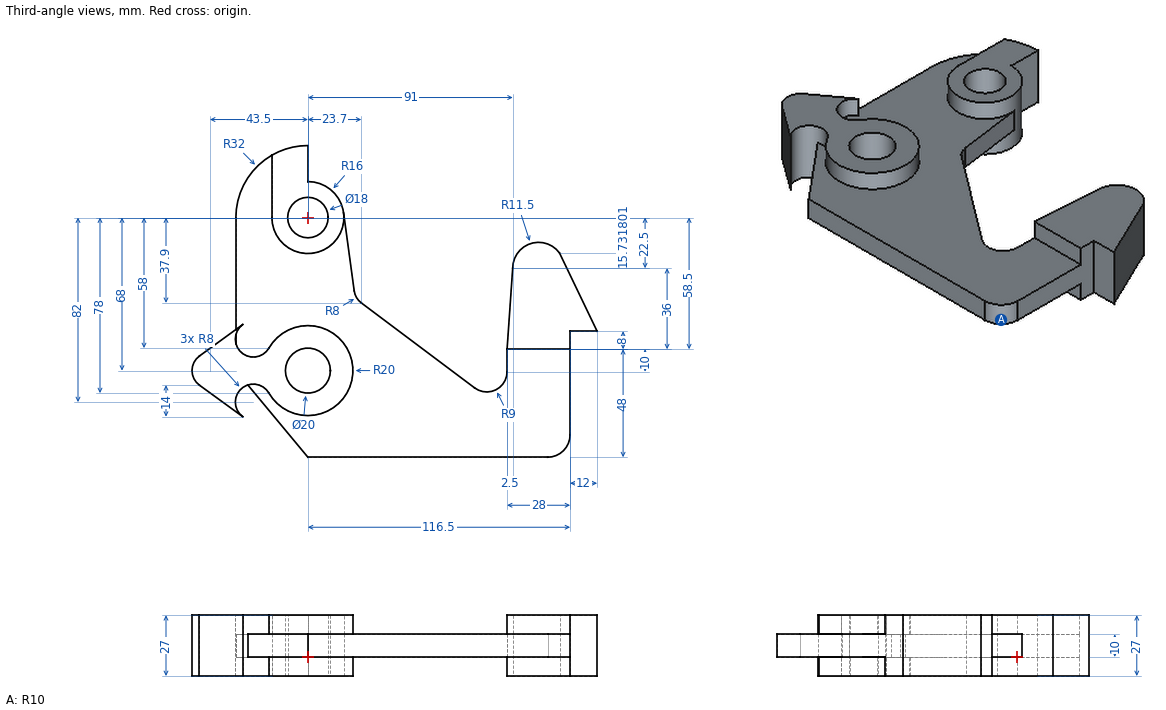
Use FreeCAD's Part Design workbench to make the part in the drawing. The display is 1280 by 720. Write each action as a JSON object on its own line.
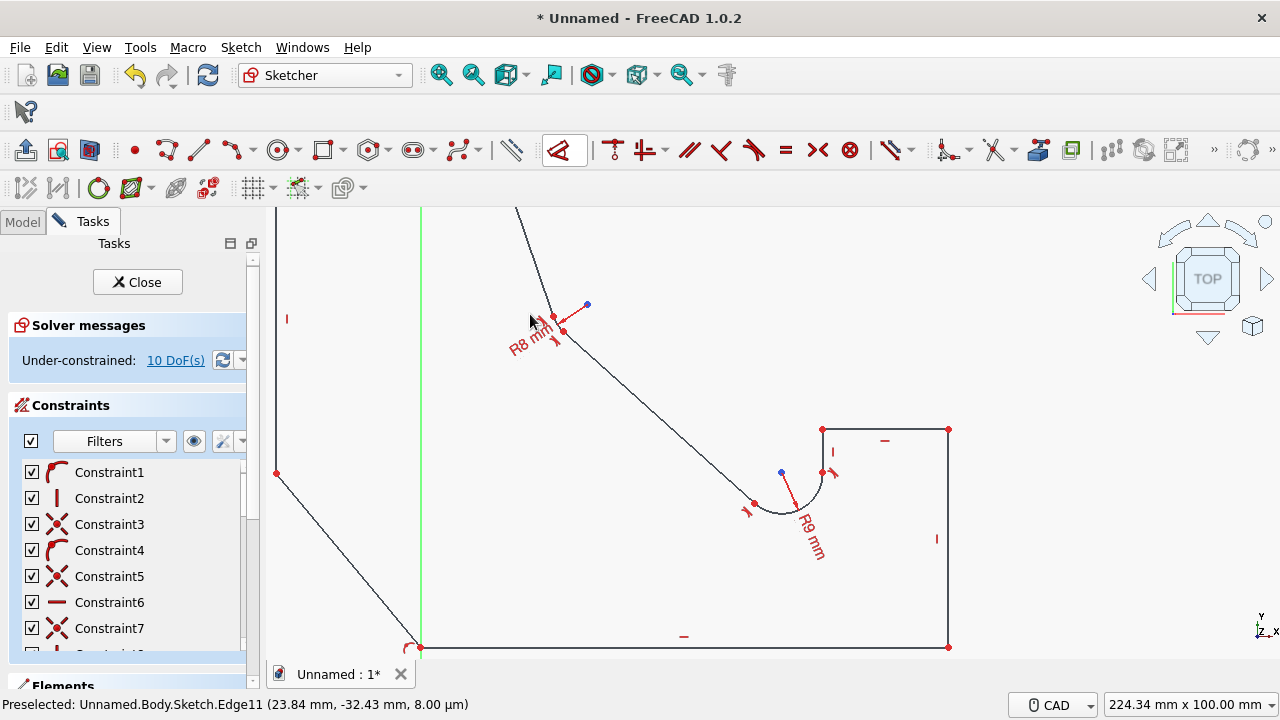
{"action": "scroll", "coordinate": [780, 515], "scroll_direction": "down", "scroll_amount": 4}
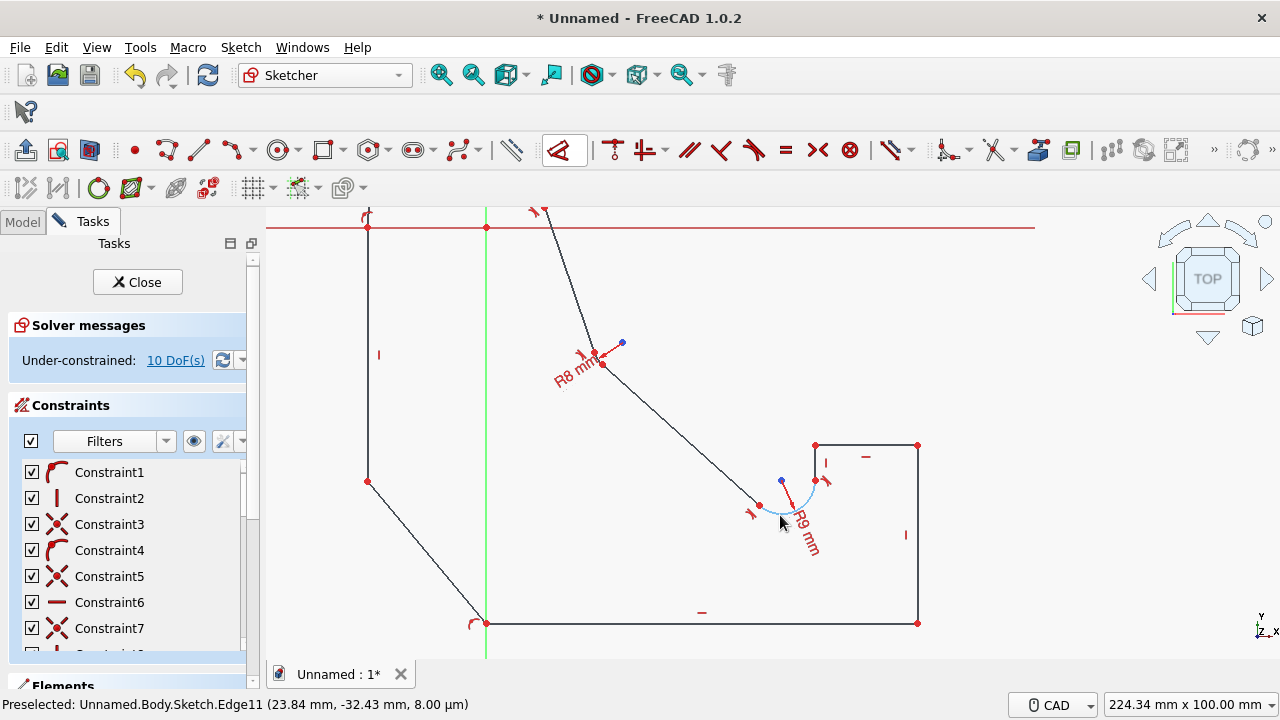
{"action": "scroll", "coordinate": [645, 336], "scroll_direction": "up", "scroll_amount": 2}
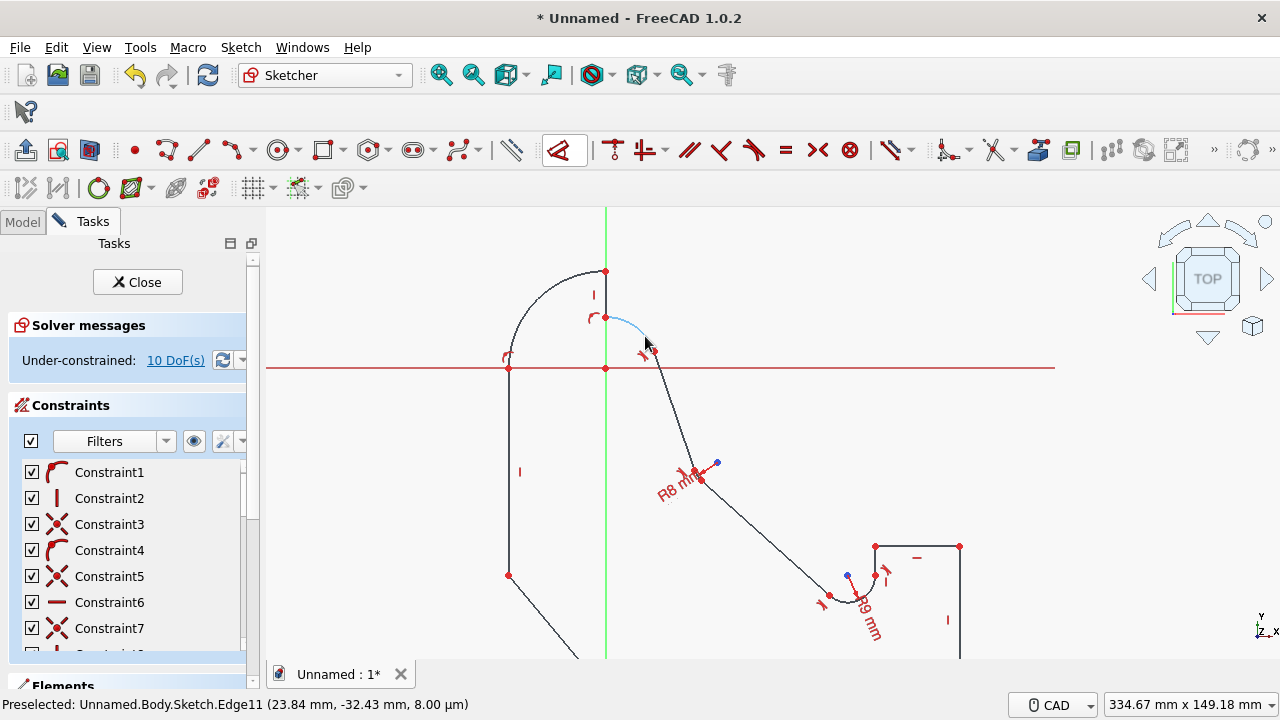
{"action": "left_click", "coordinate": [645, 335]}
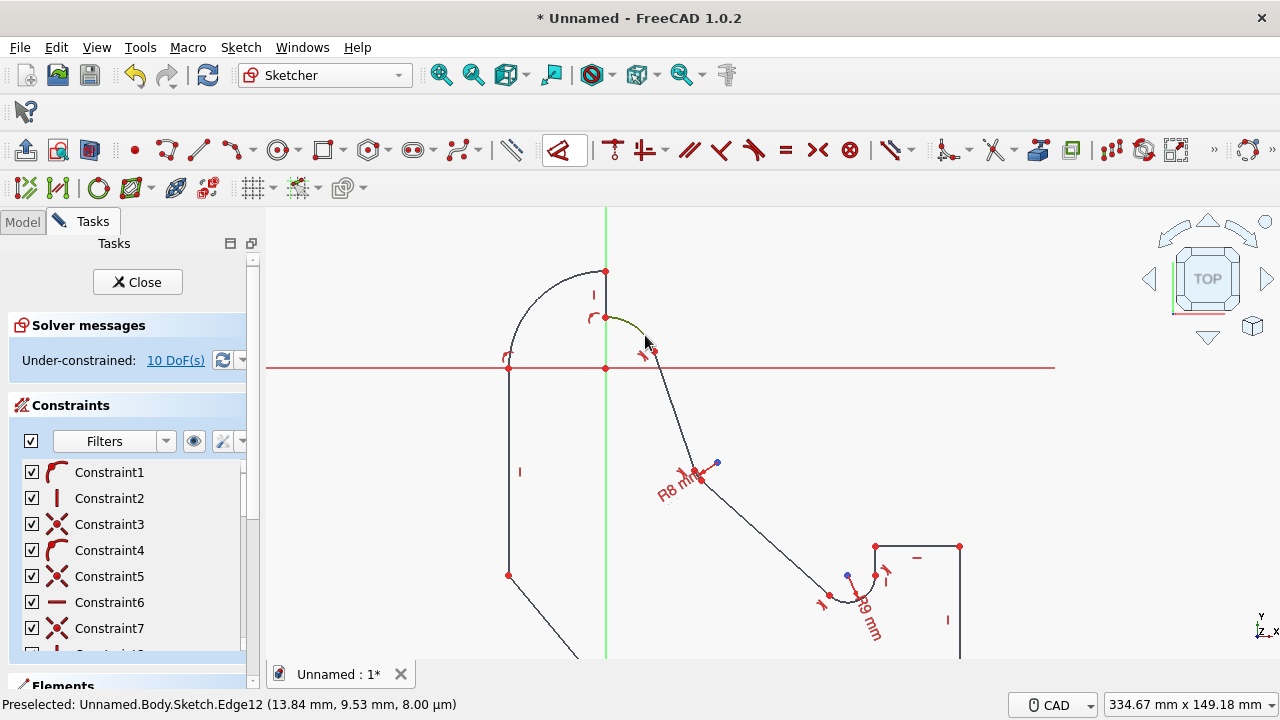
{"action": "left_click", "coordinate": [582, 150]}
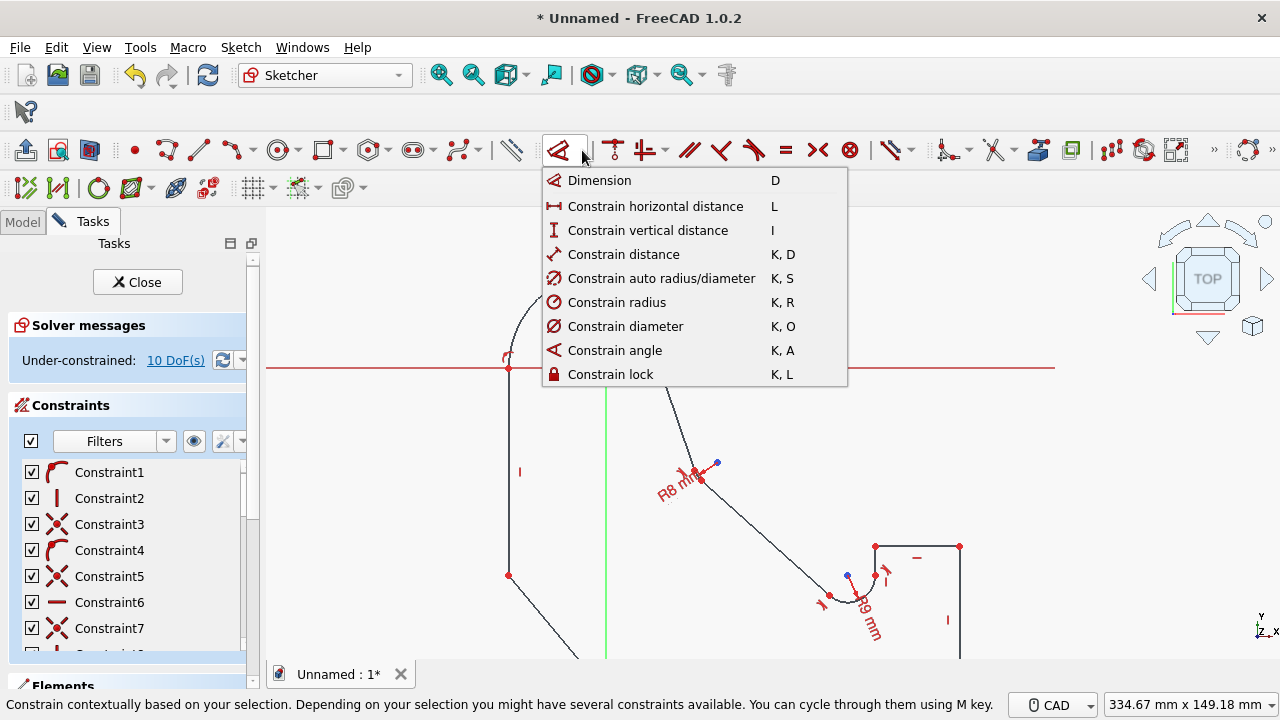
{"action": "left_click", "coordinate": [695, 302]}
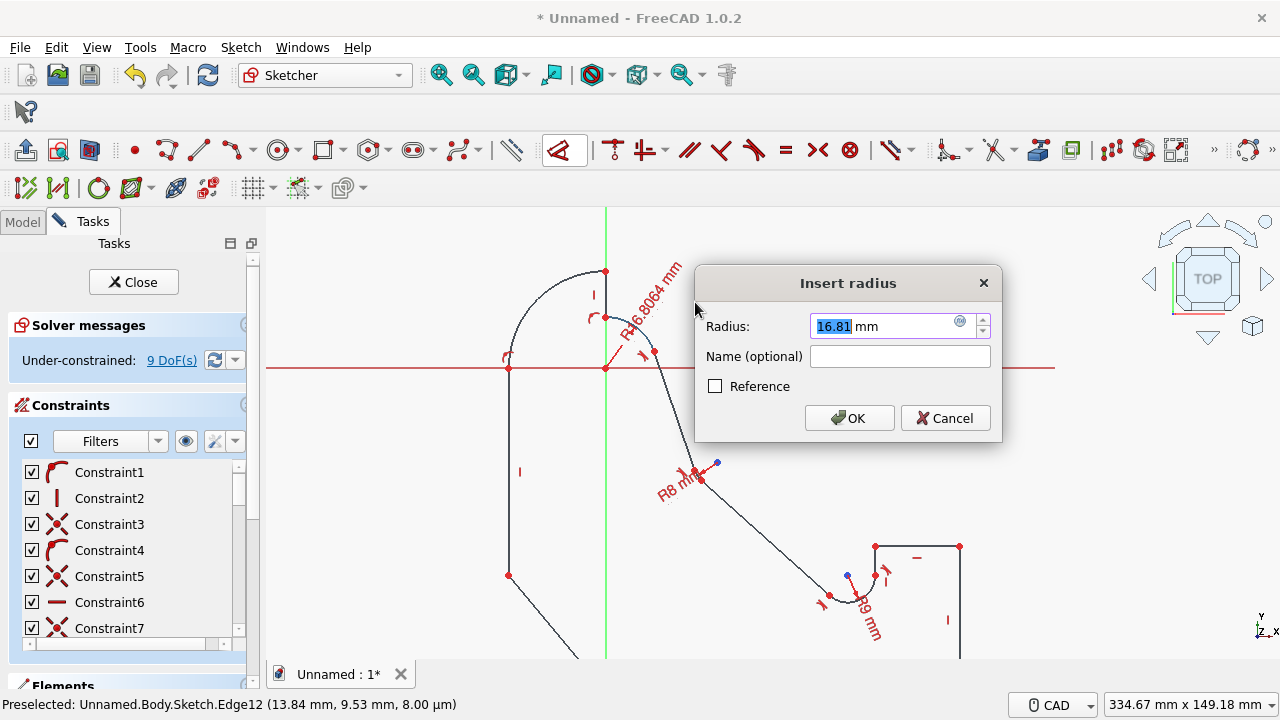
{"action": "type", "text": "16"}
{"action": "key", "text": "Return"}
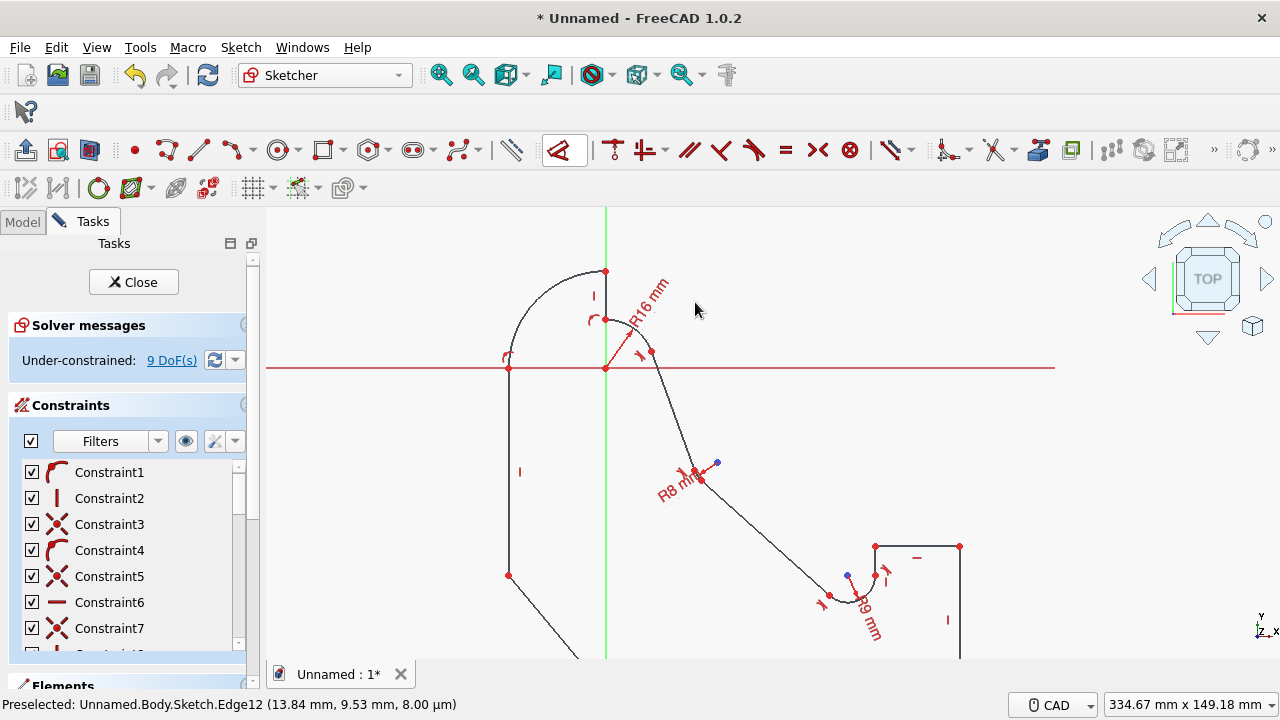
{"action": "left_click", "coordinate": [562, 282]}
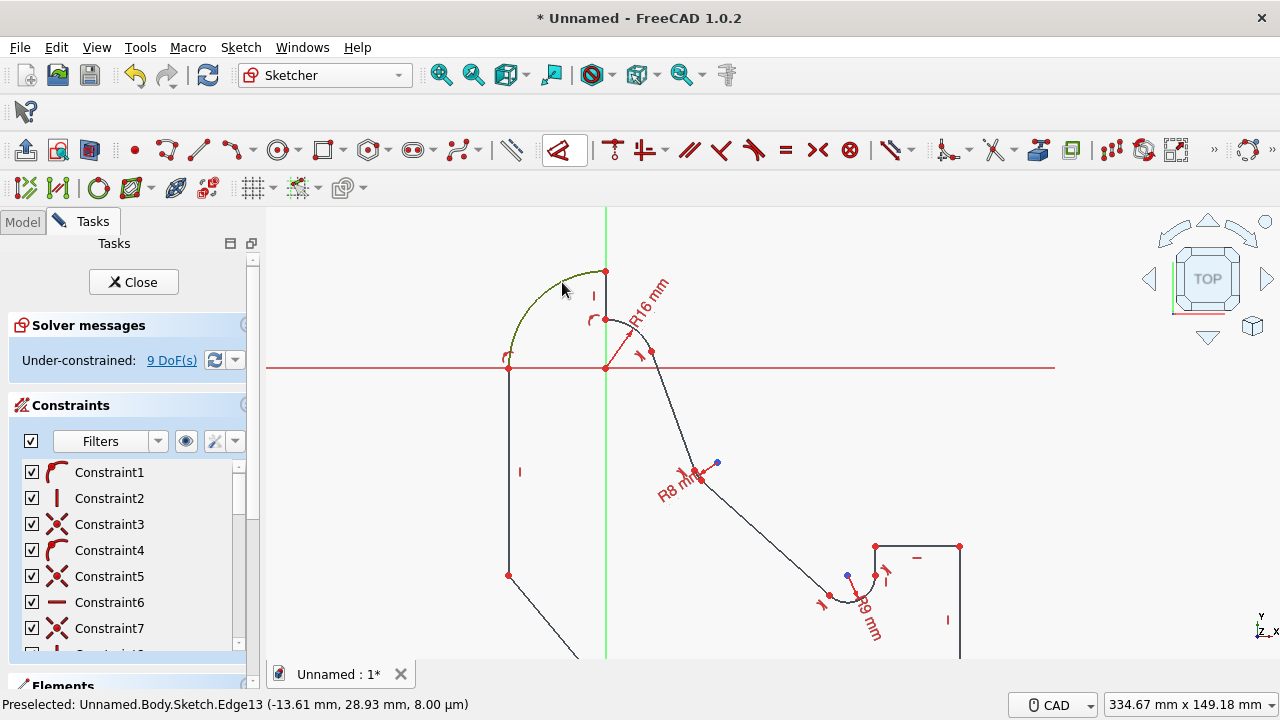
{"action": "left_click", "coordinate": [582, 150]}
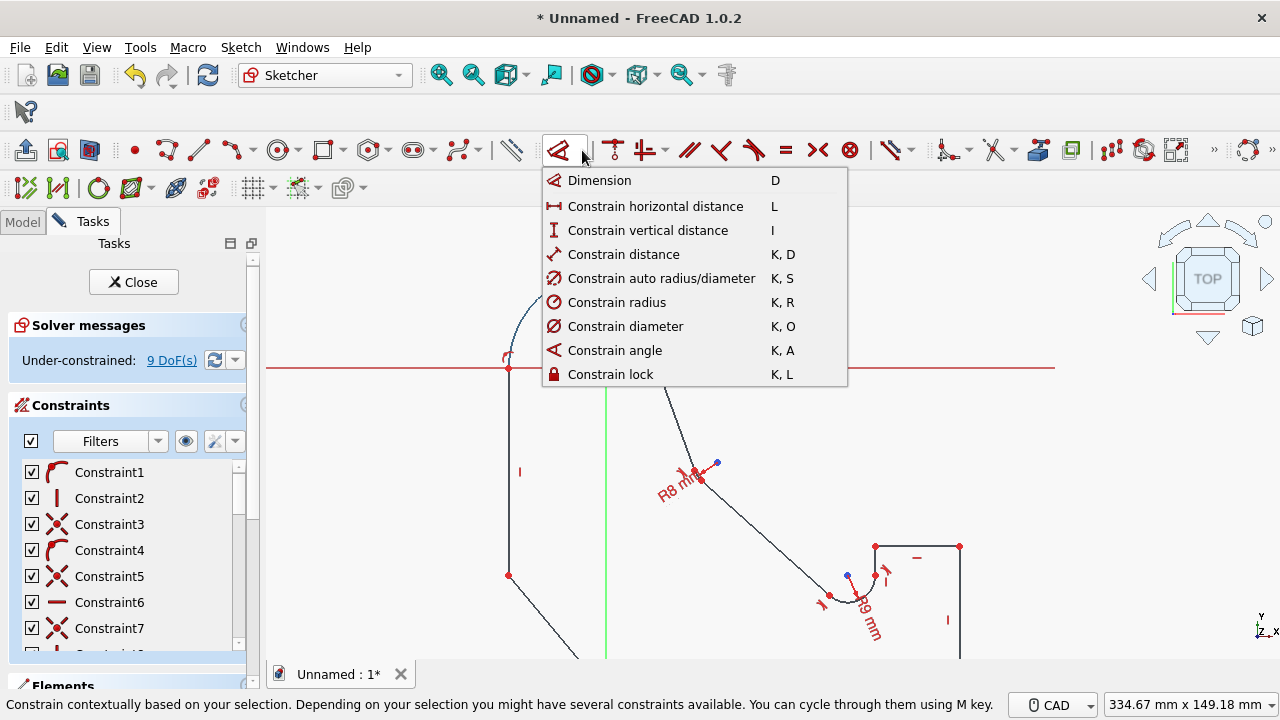
{"action": "left_click", "coordinate": [695, 302]}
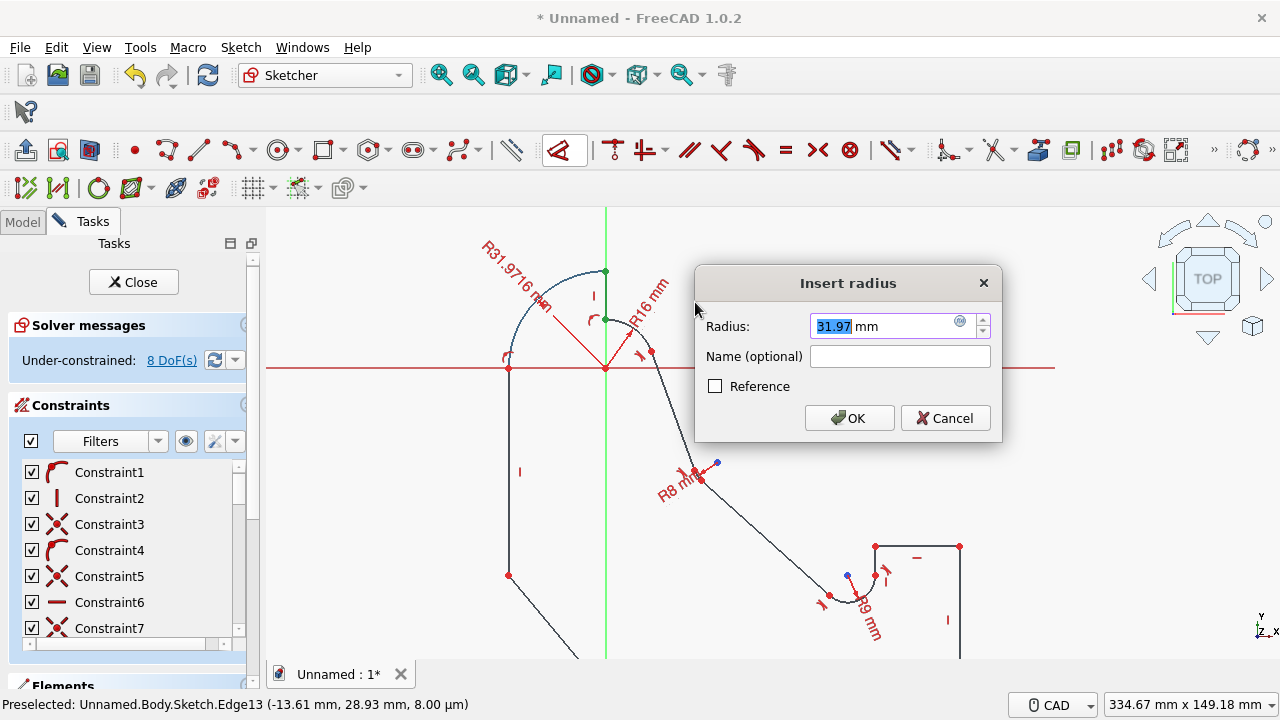
{"action": "type", "text": "32"}
{"action": "key", "text": "Return"}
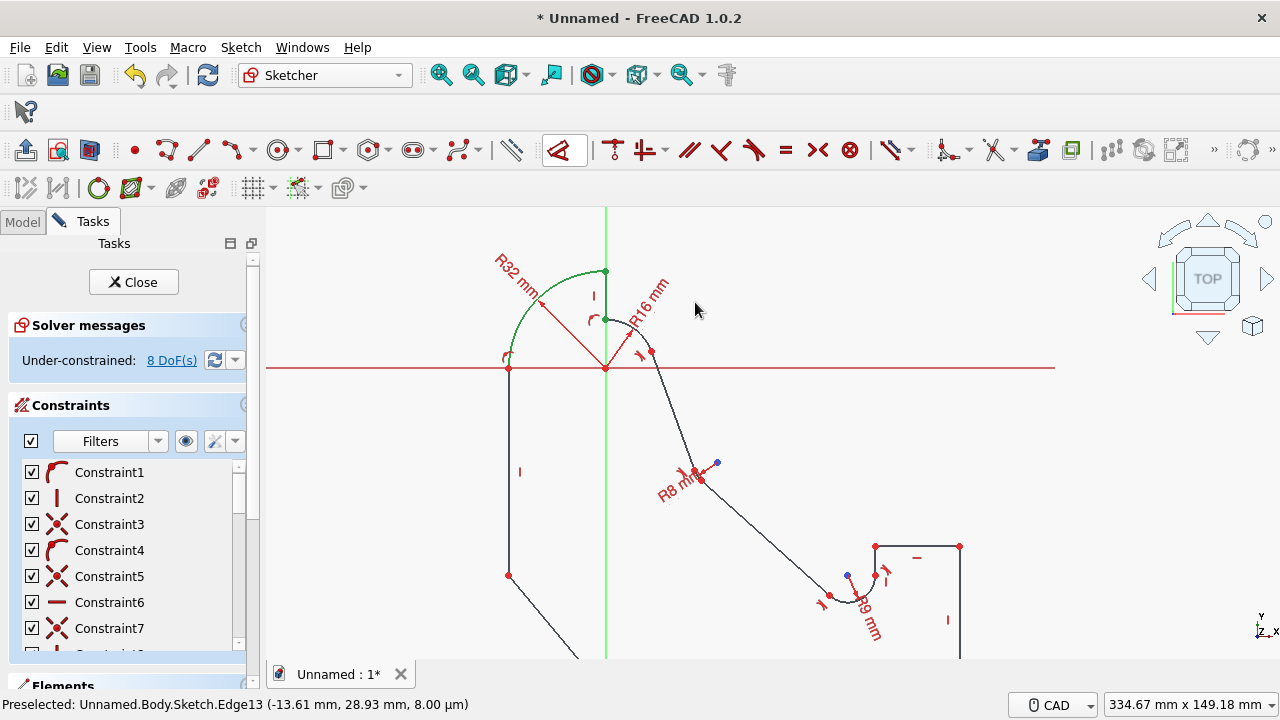
{"action": "left_click", "coordinate": [509, 430]}